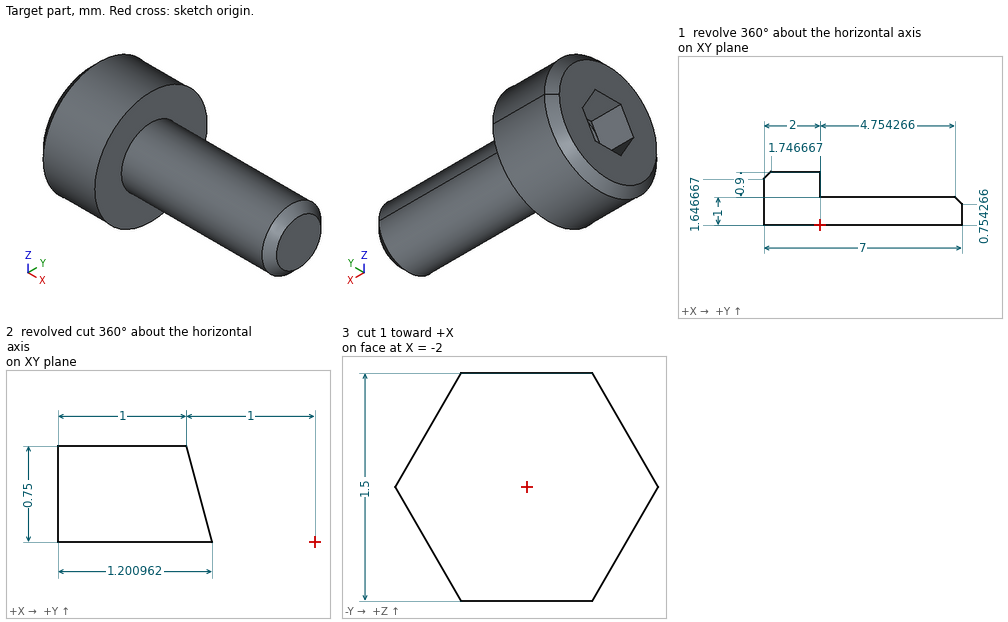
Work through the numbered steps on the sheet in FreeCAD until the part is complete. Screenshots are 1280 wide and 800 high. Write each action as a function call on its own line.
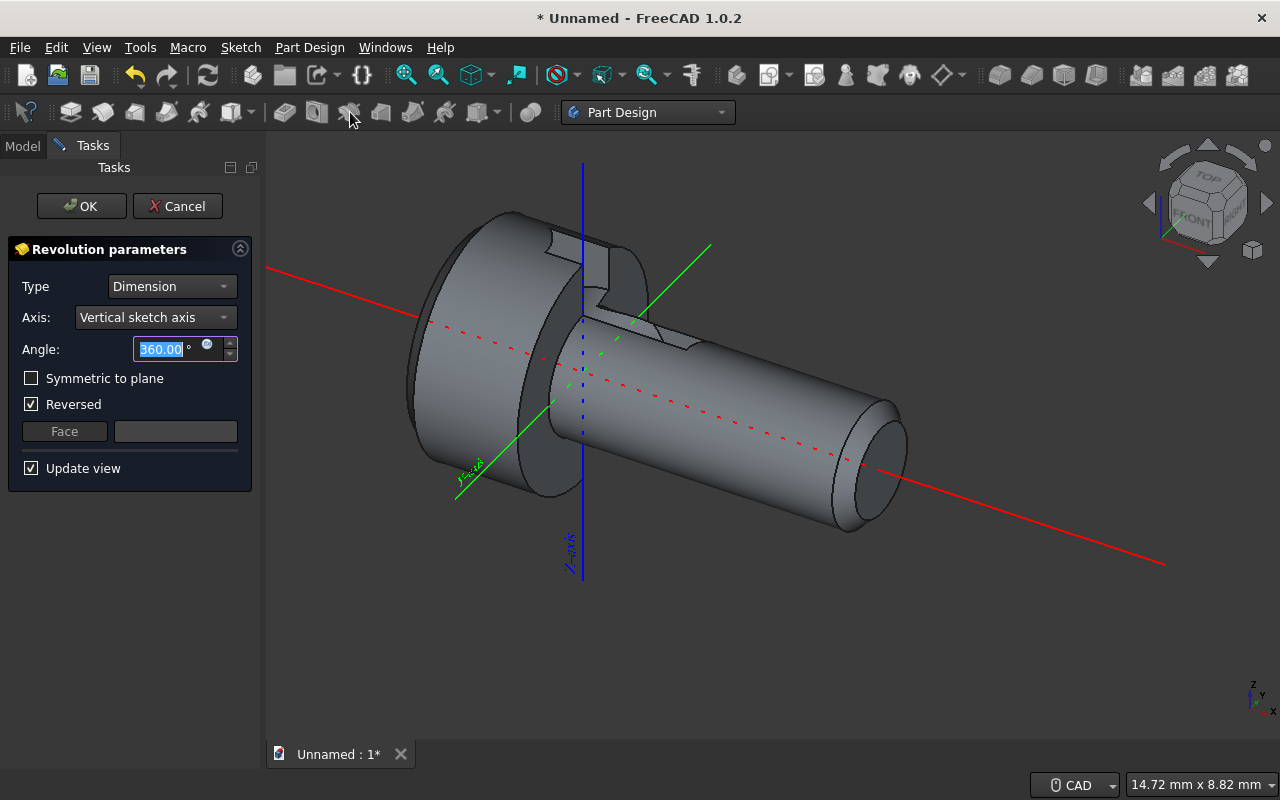
click(156, 318)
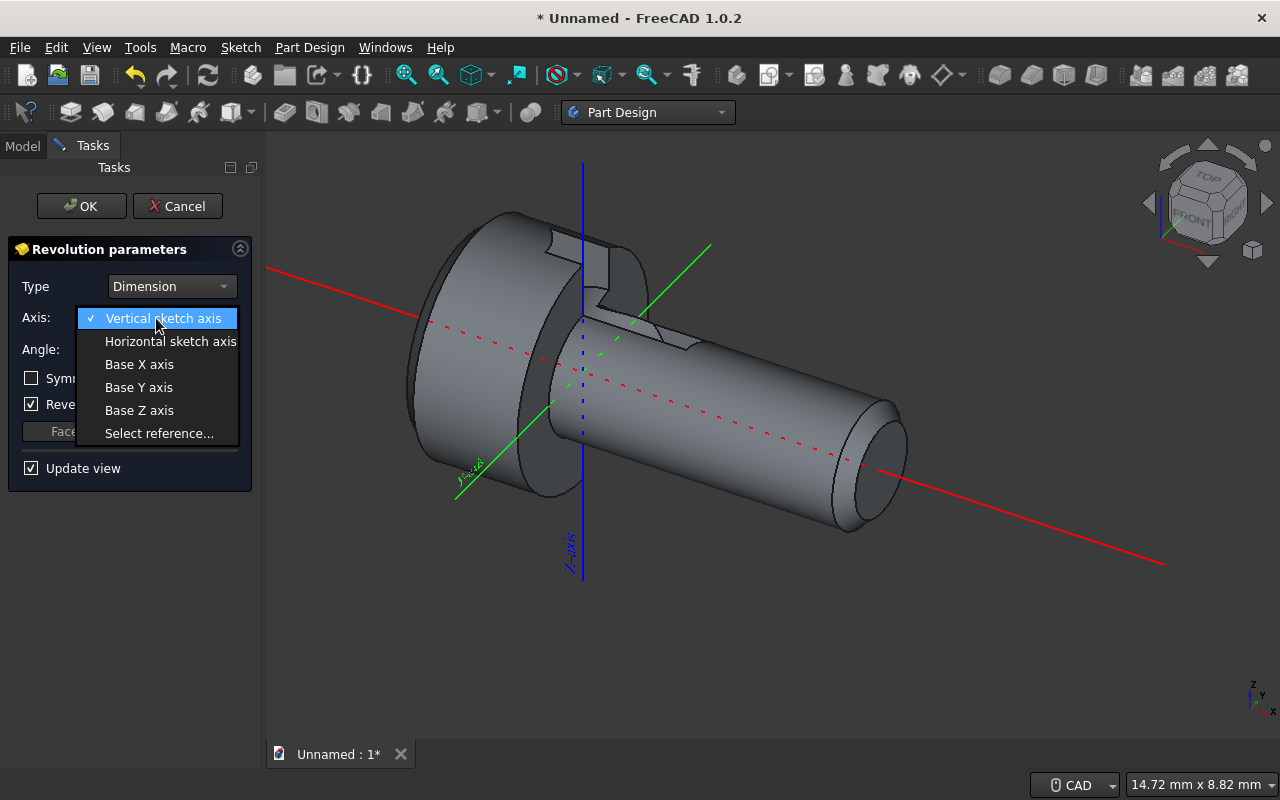
click(156, 342)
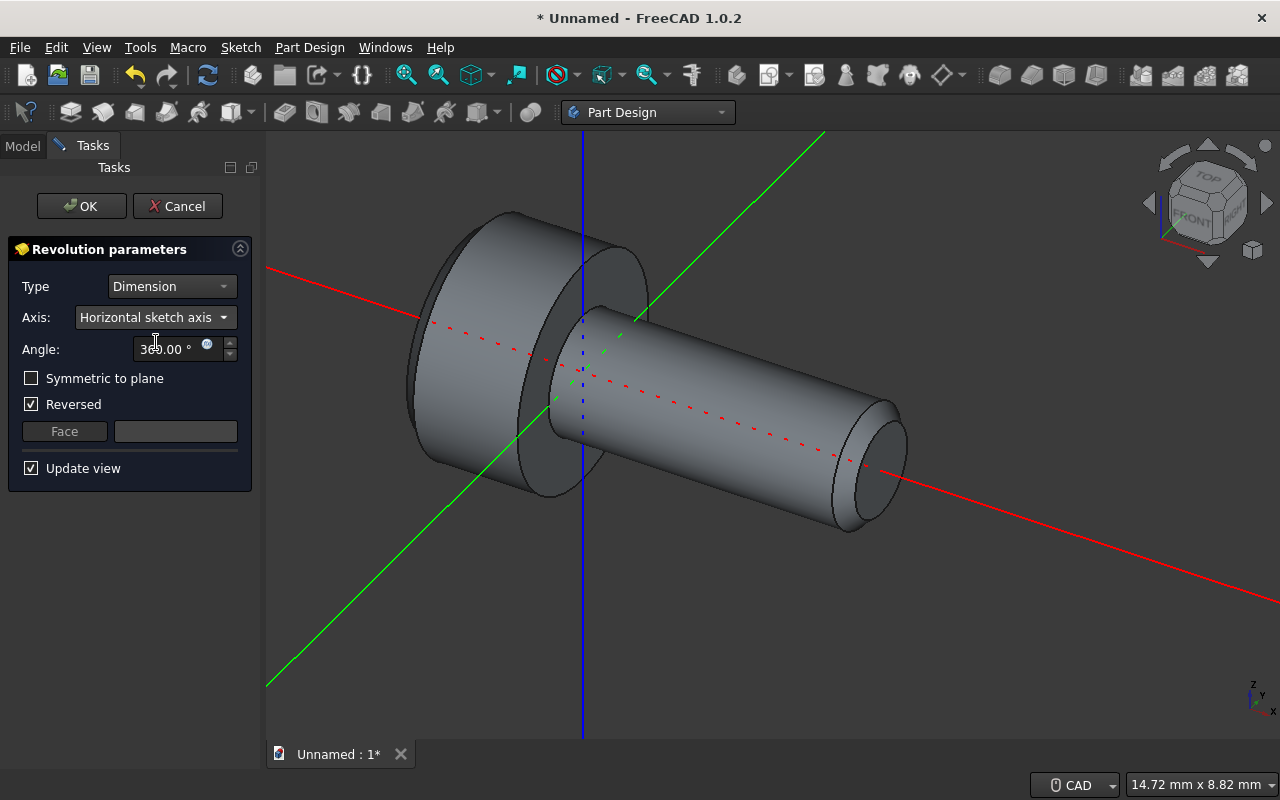
click(82, 206)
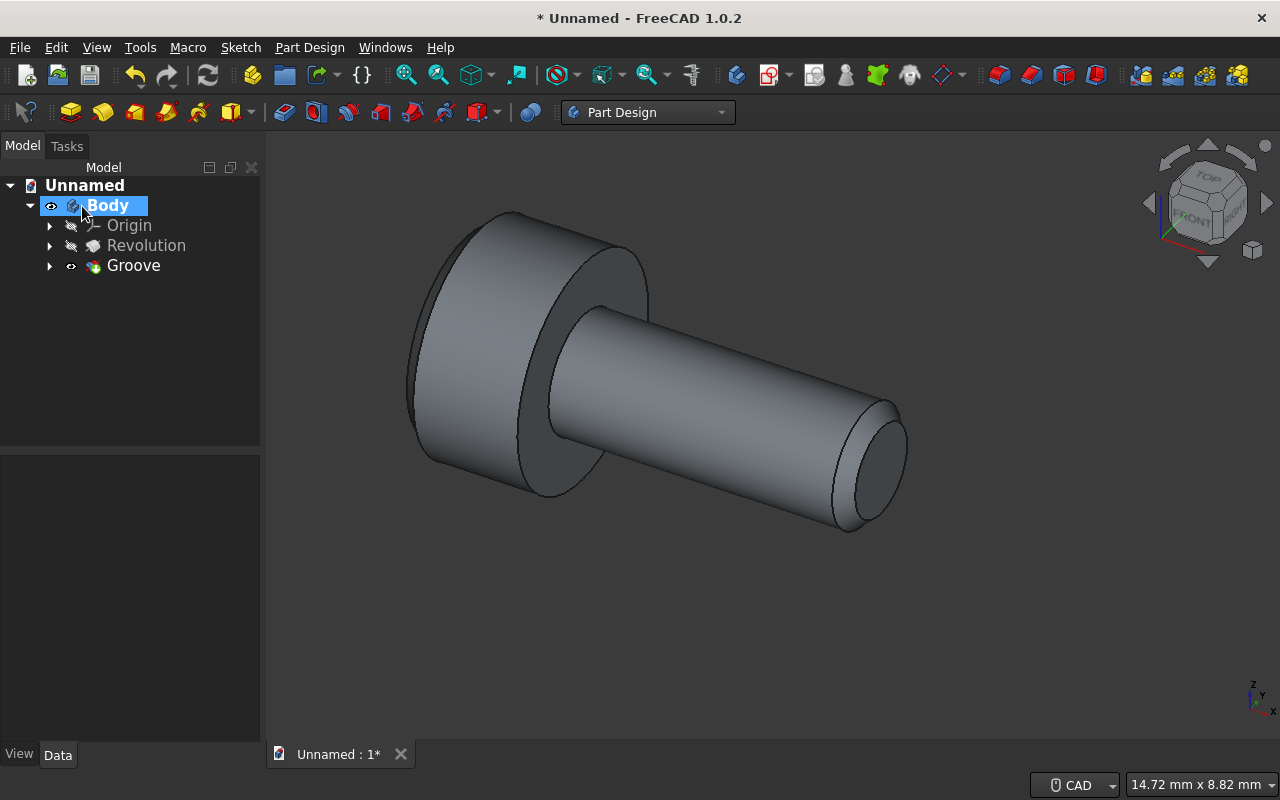
key(6)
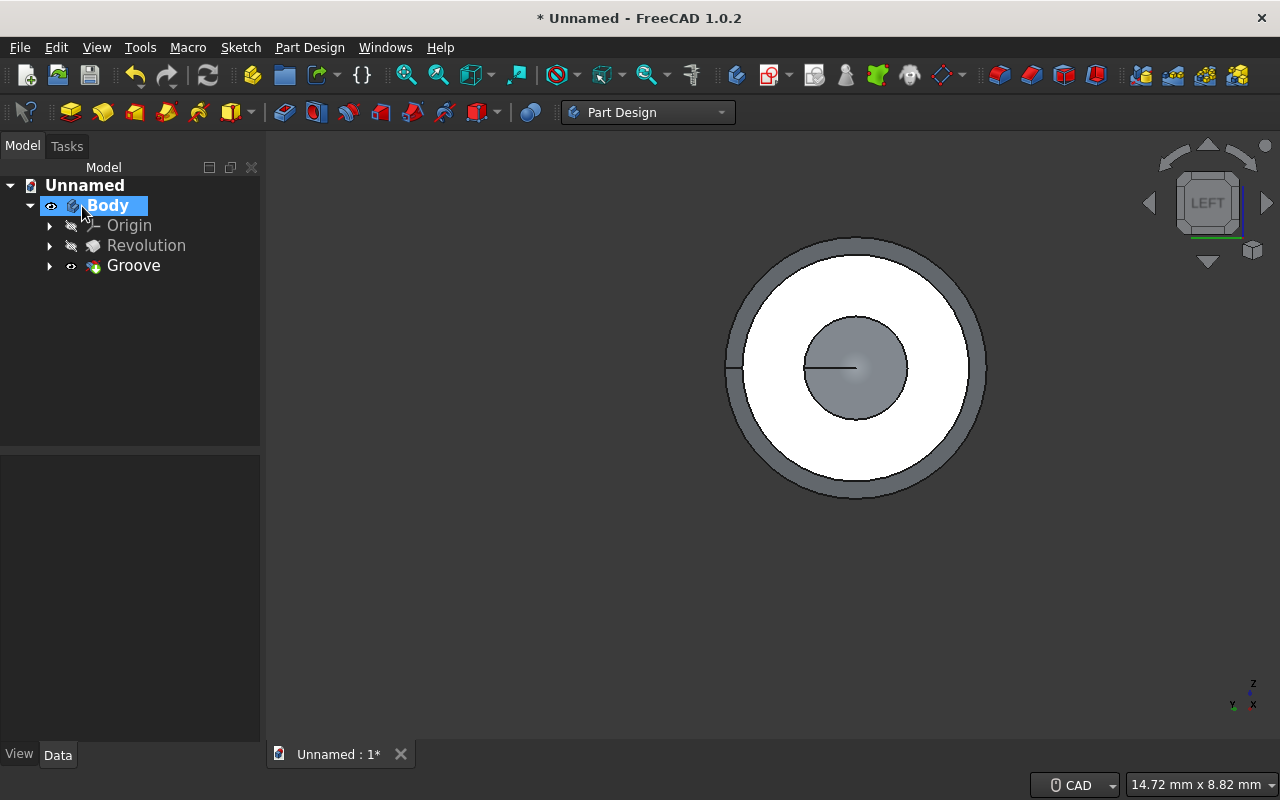
click(408, 76)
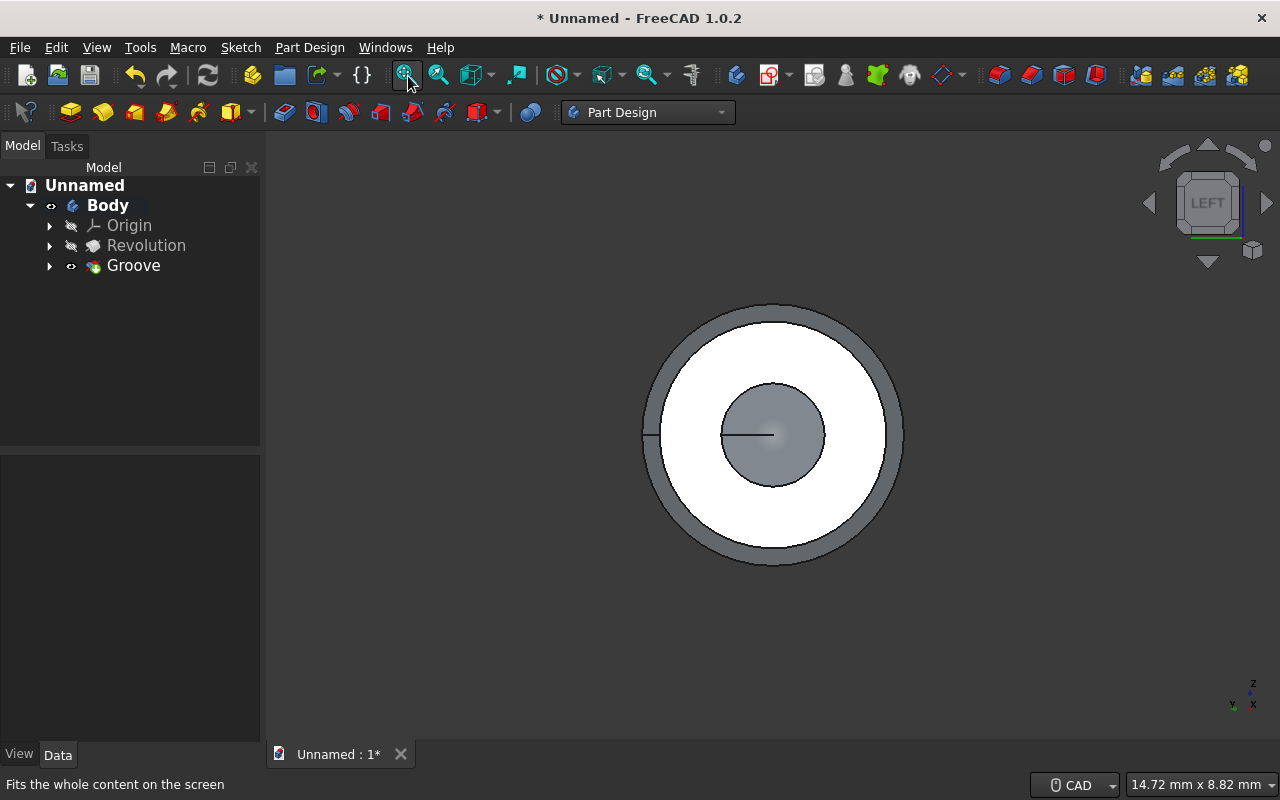
click(838, 499)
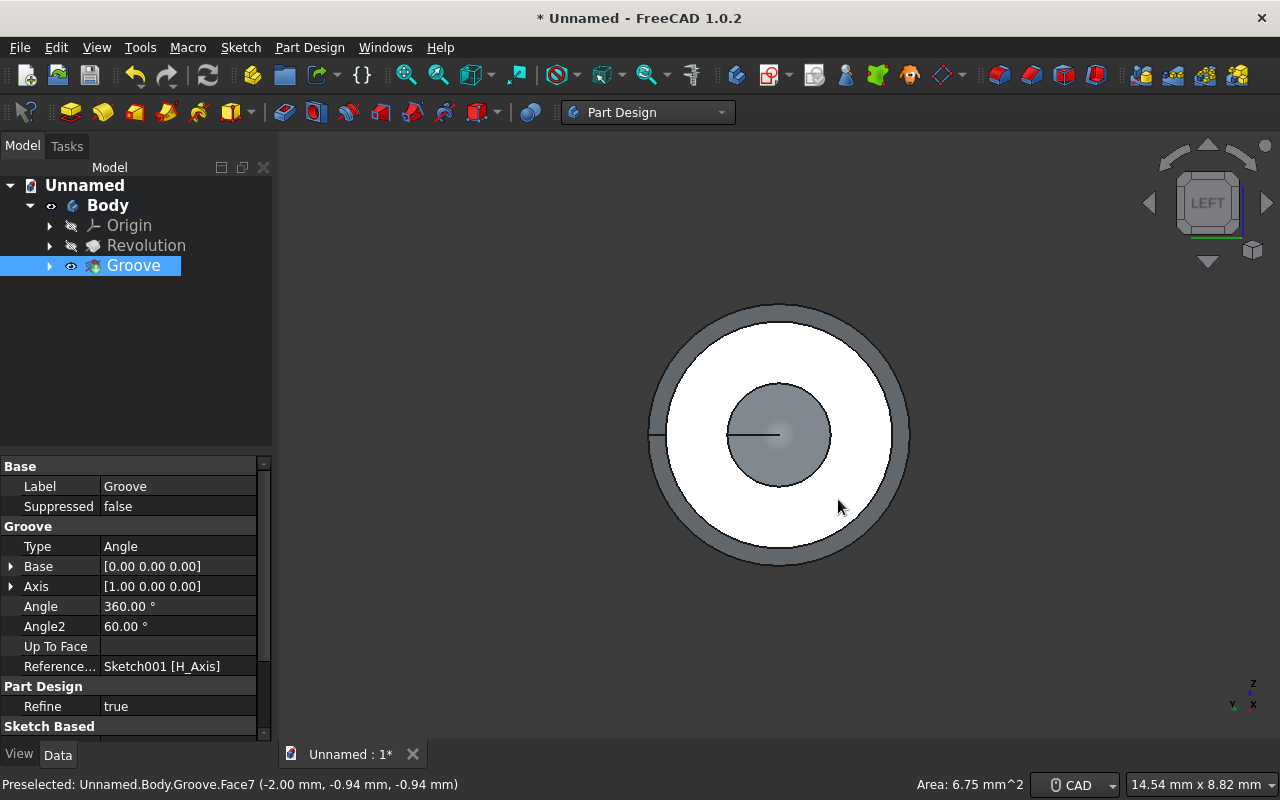
click(770, 76)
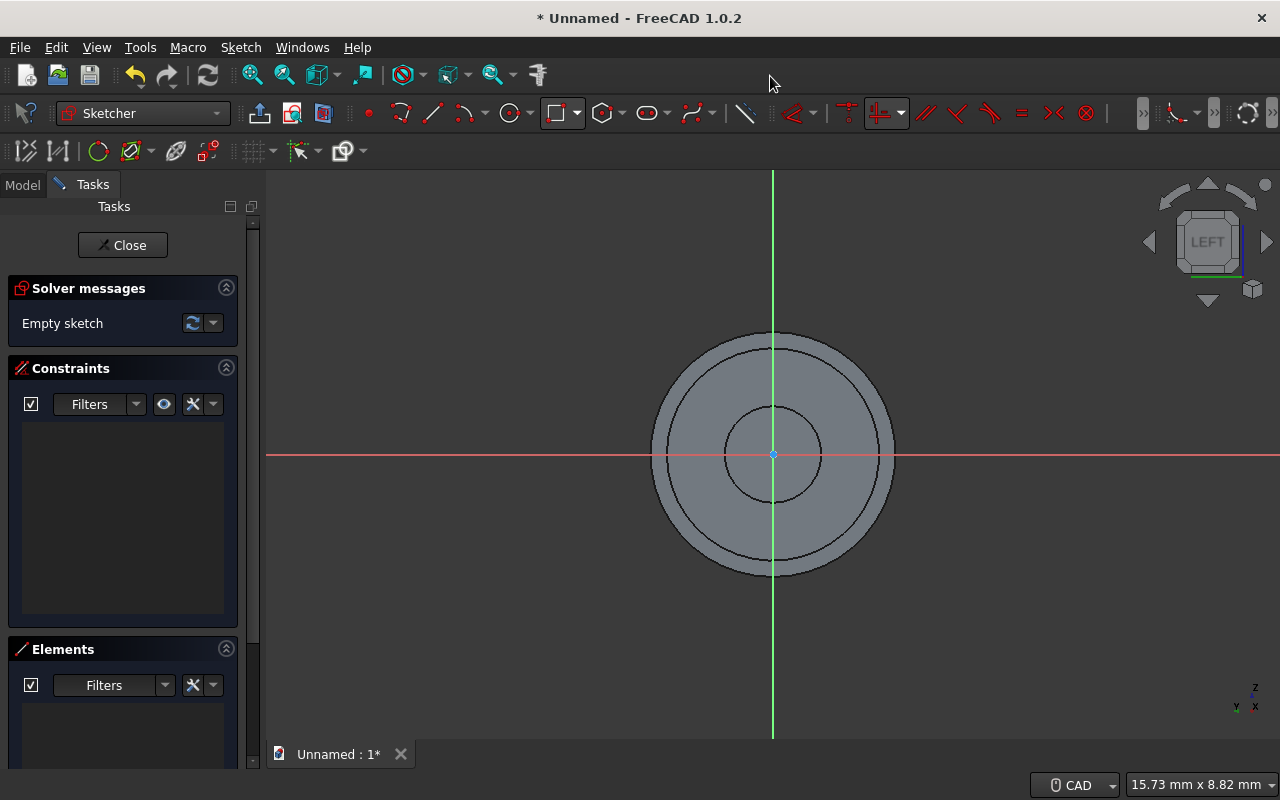
scroll(795, 454, up, 7)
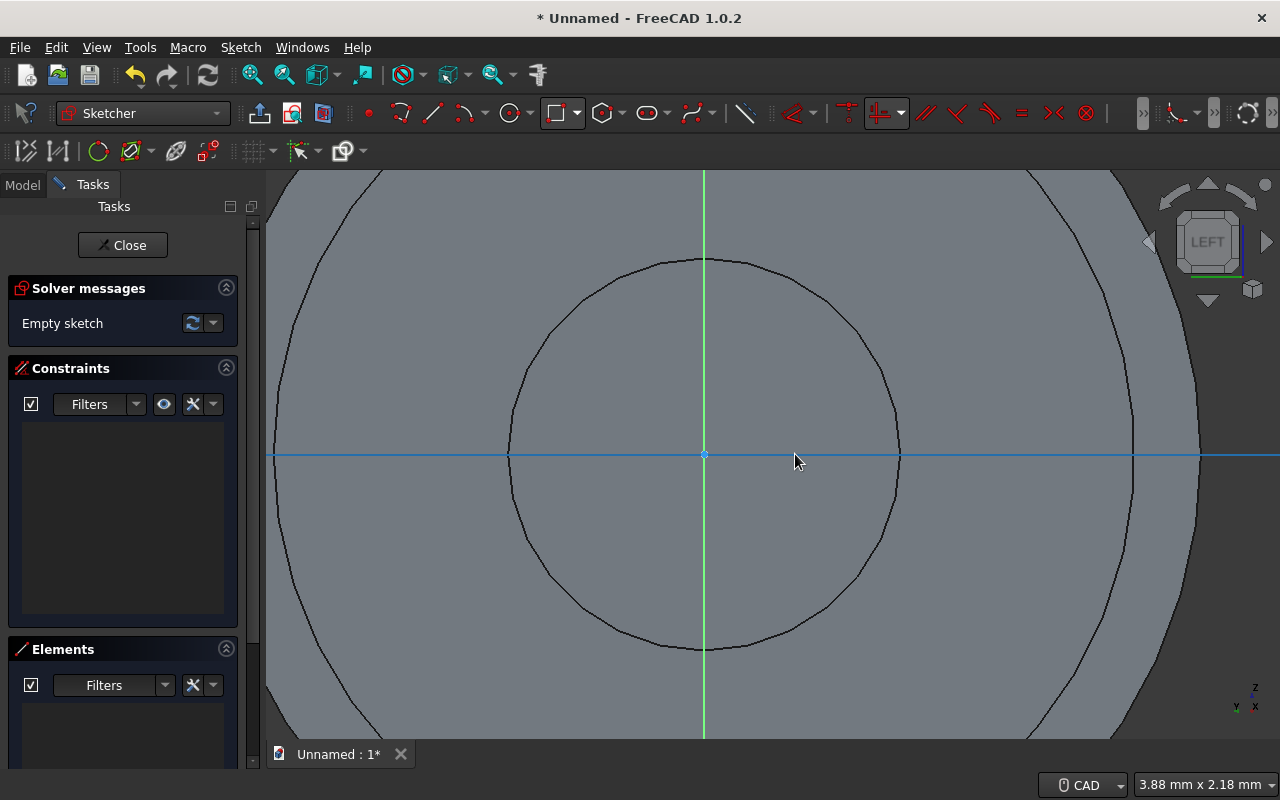
click(602, 114)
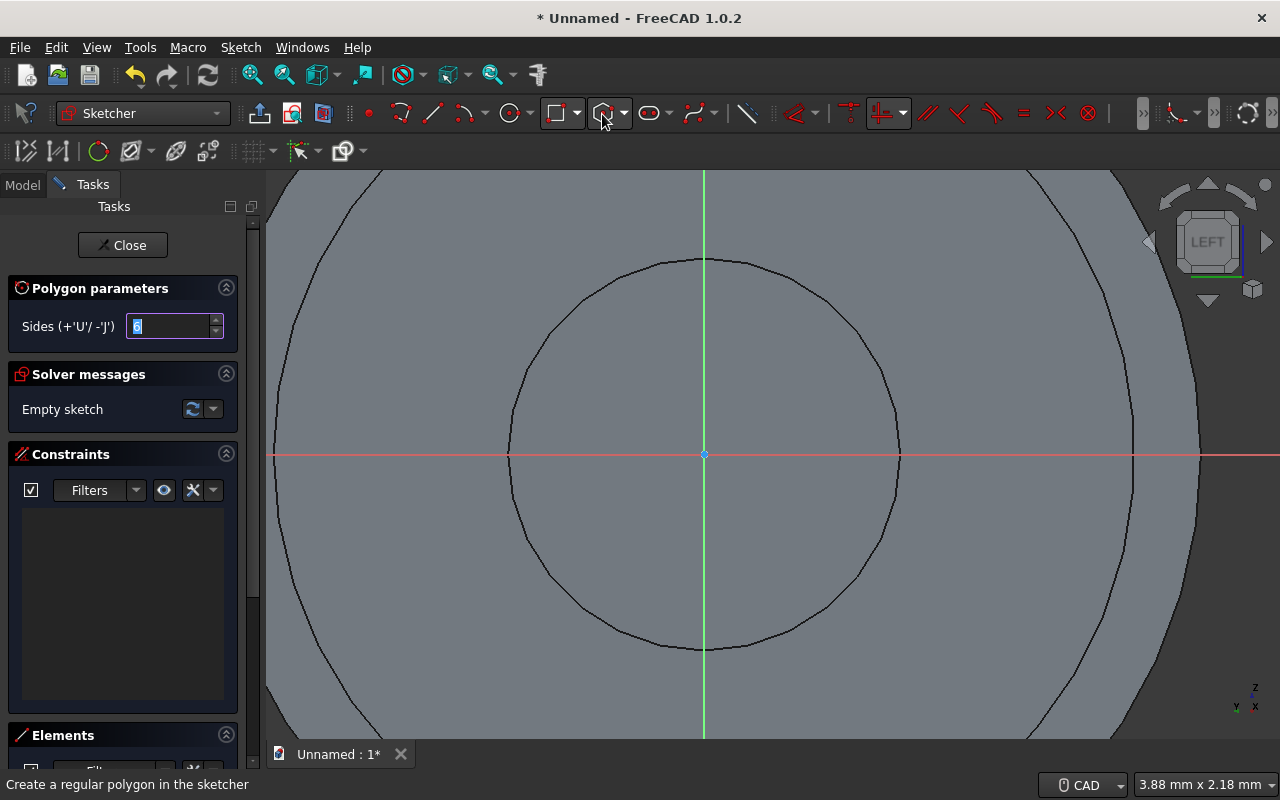
click(704, 454)